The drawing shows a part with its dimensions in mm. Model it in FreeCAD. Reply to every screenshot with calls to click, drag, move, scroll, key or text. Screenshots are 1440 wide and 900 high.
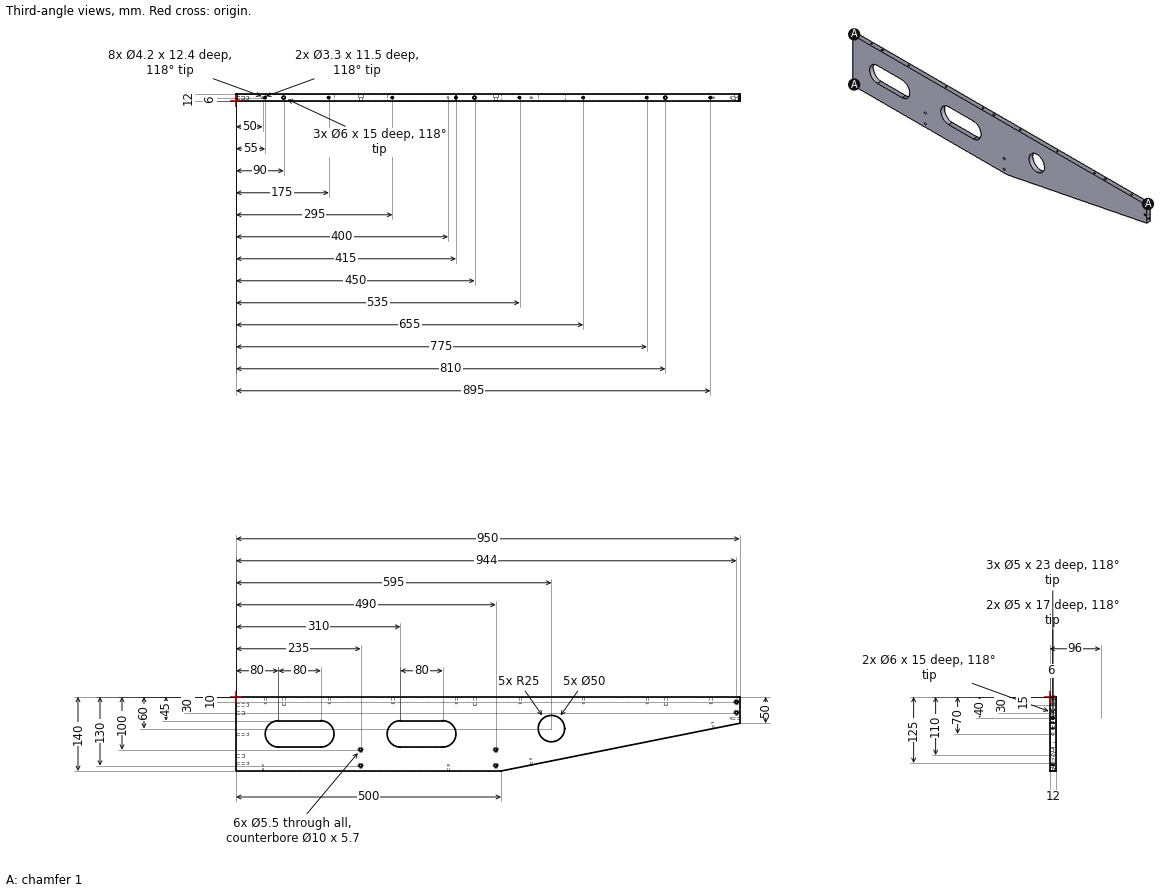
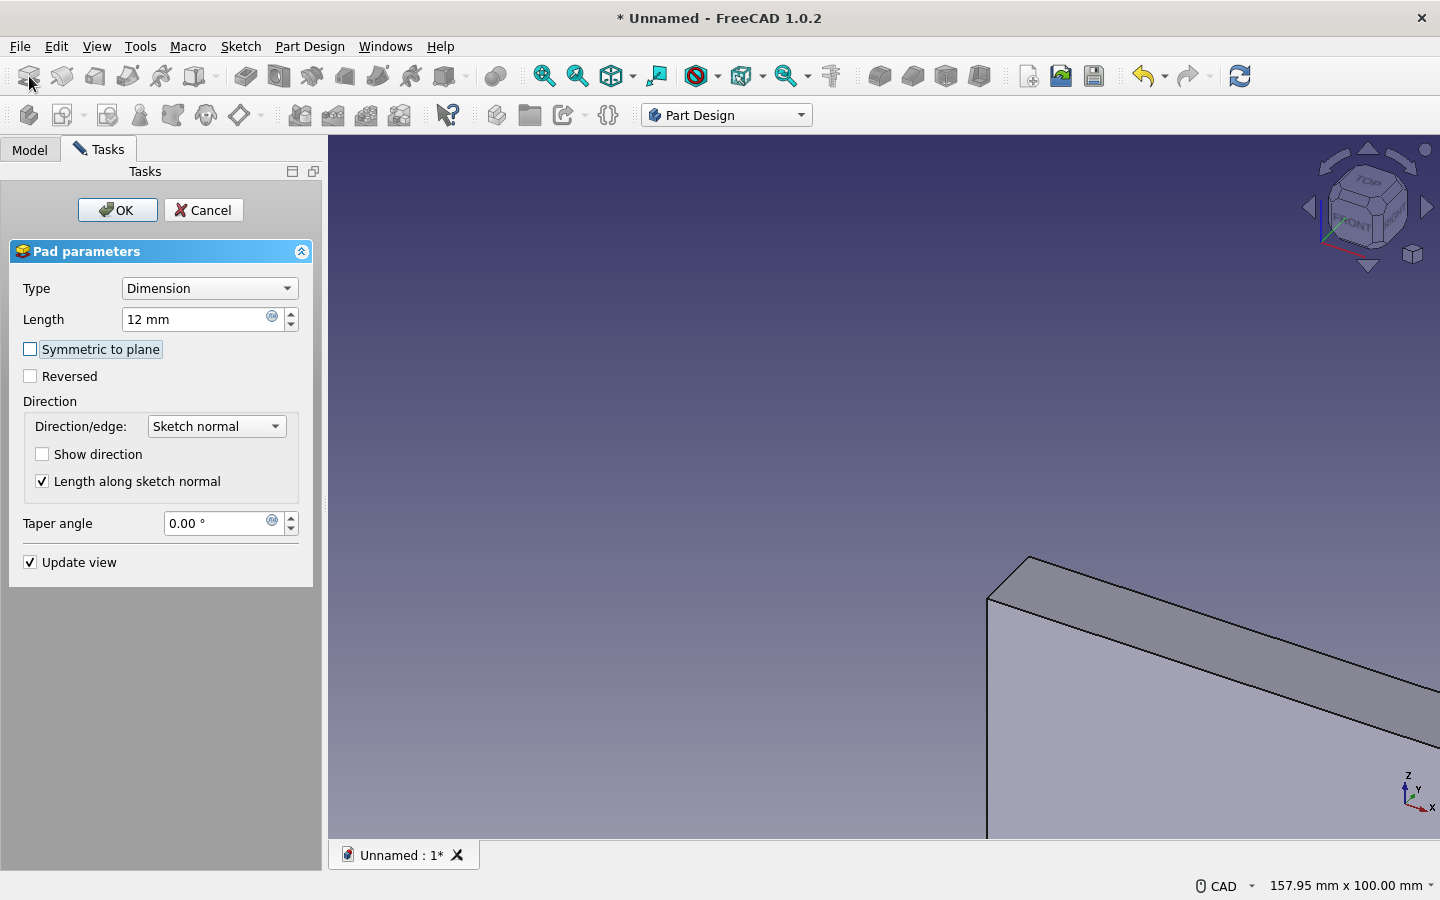
click(31, 376)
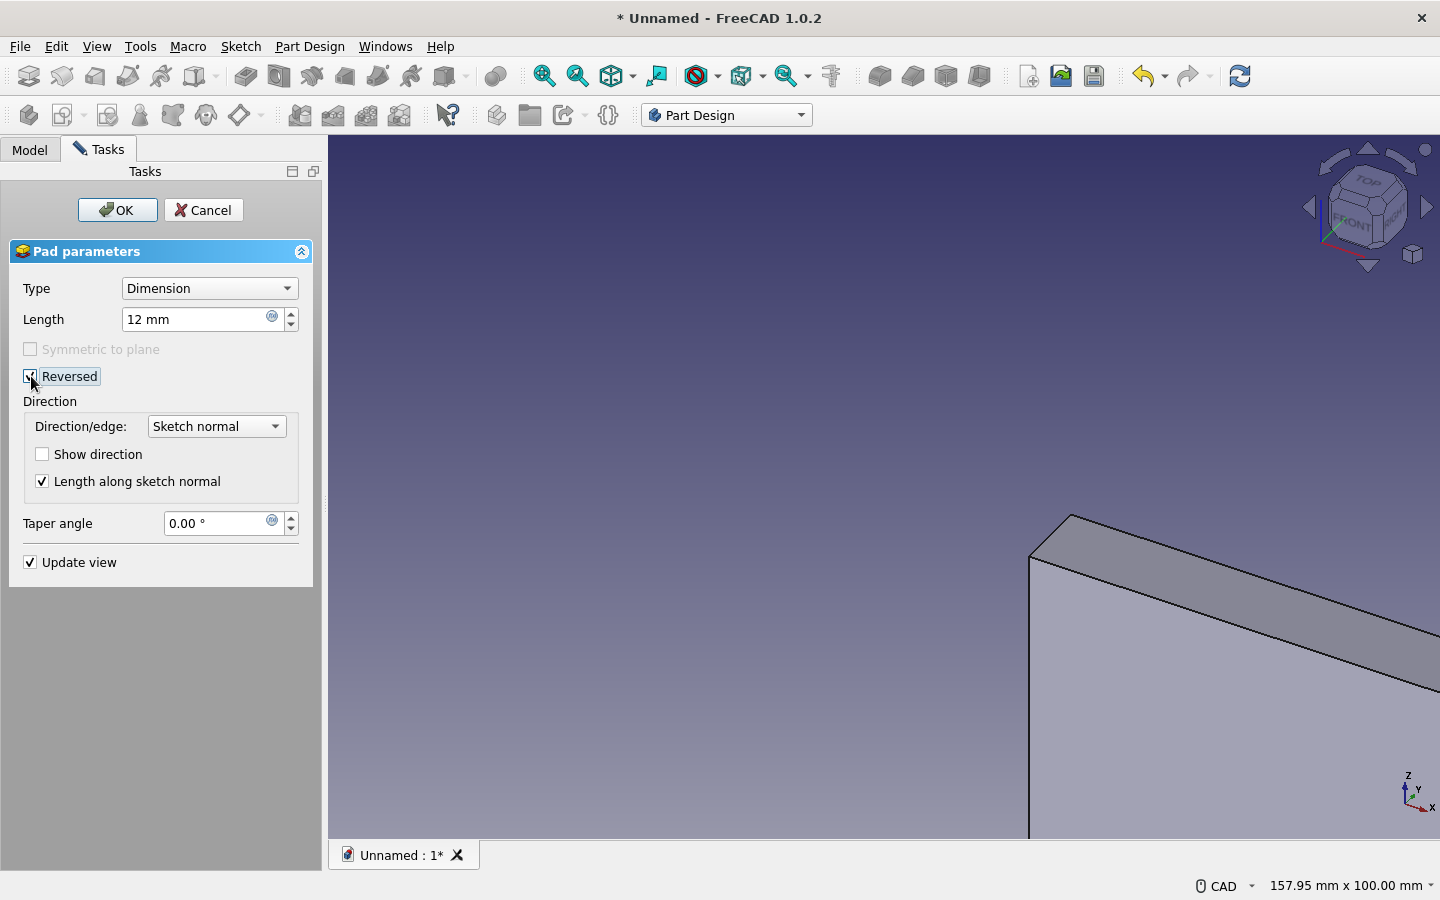
click(118, 210)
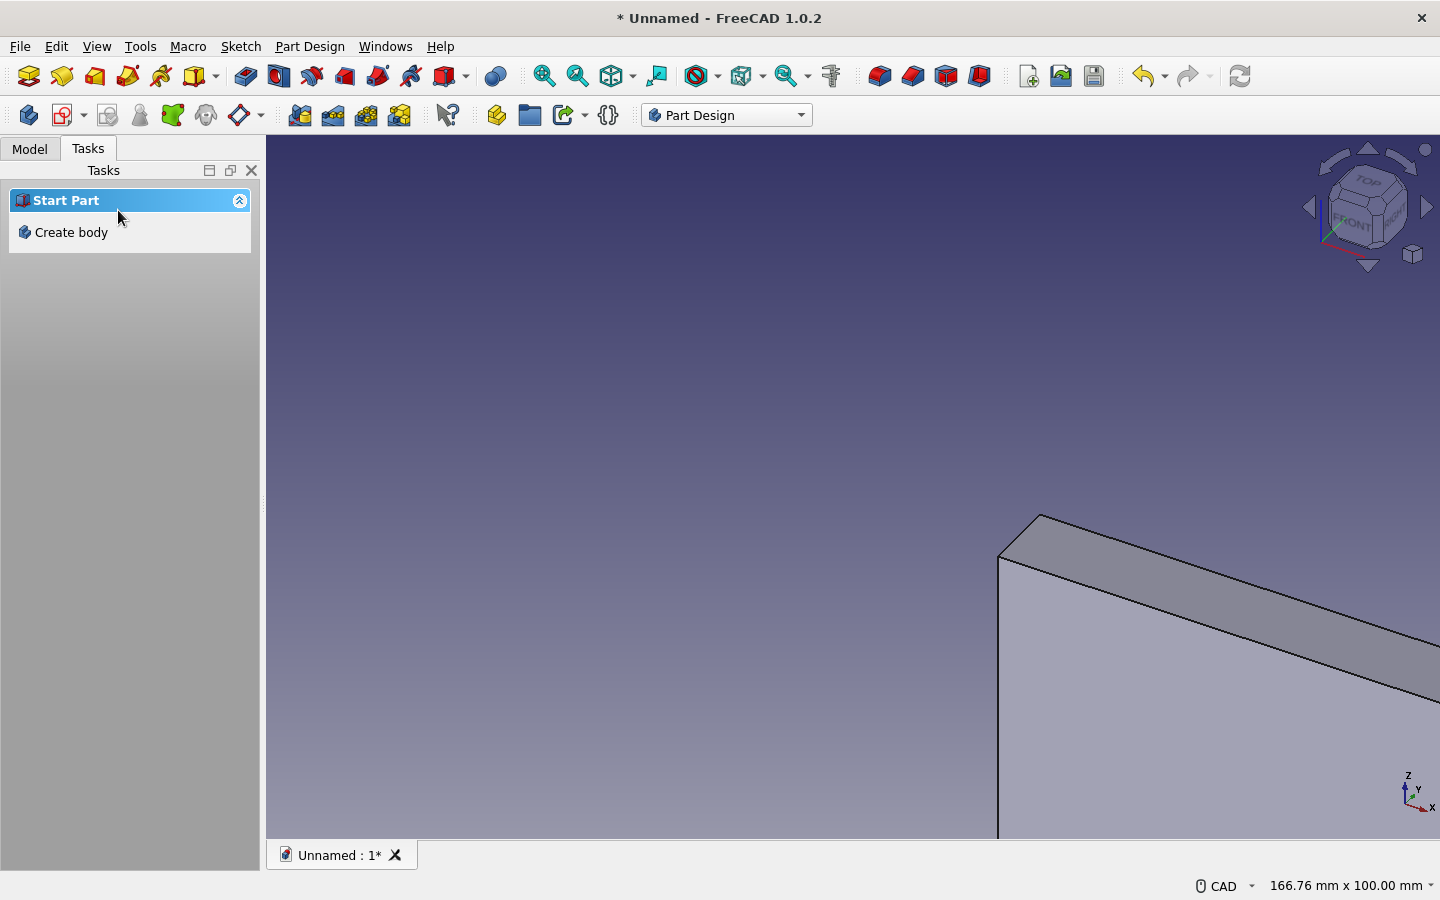
click(545, 76)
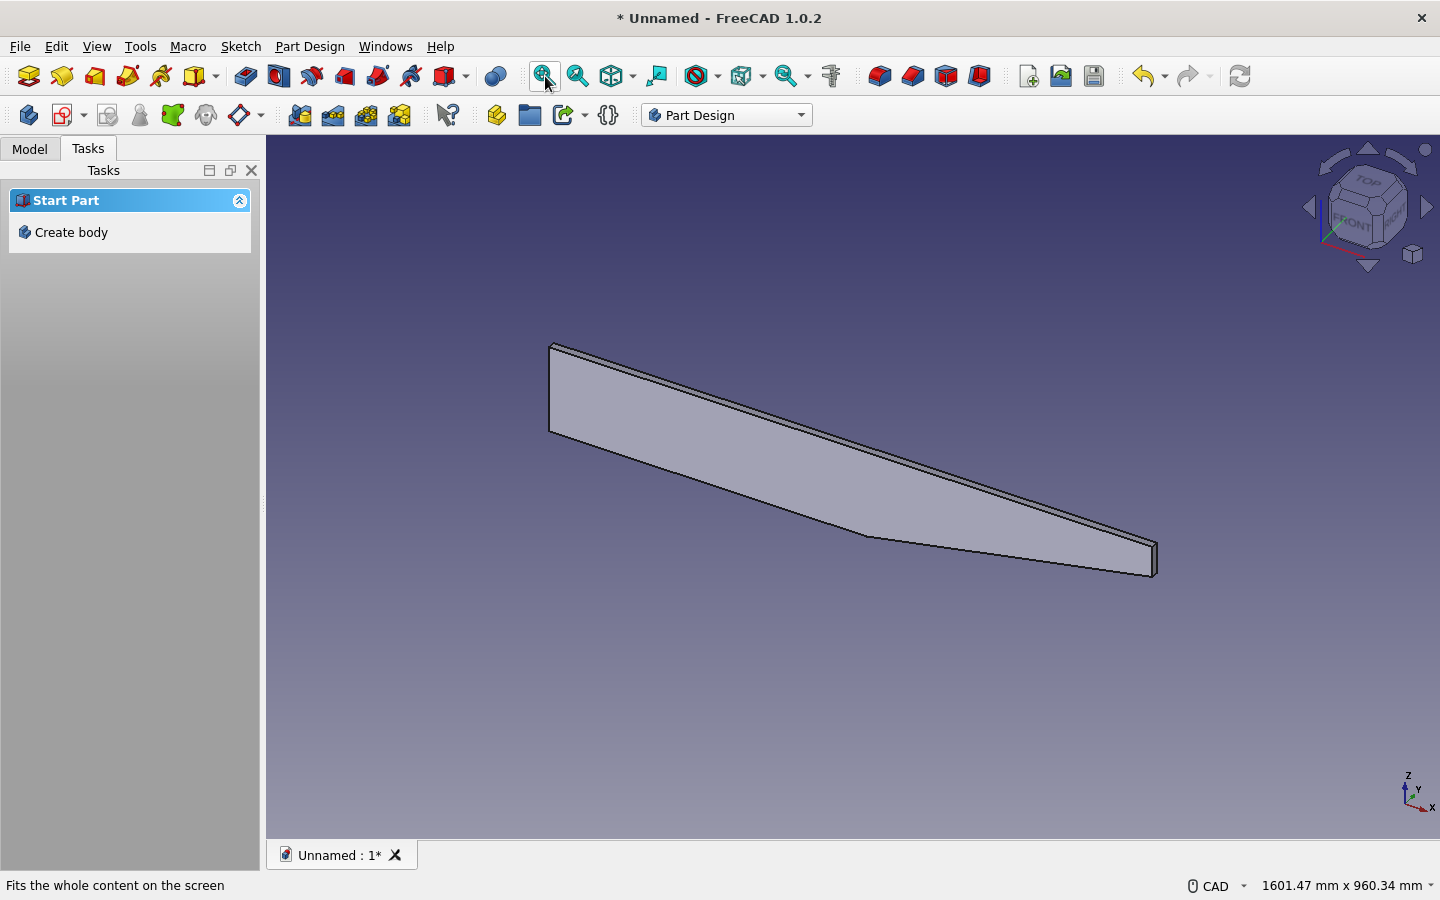
click(62, 116)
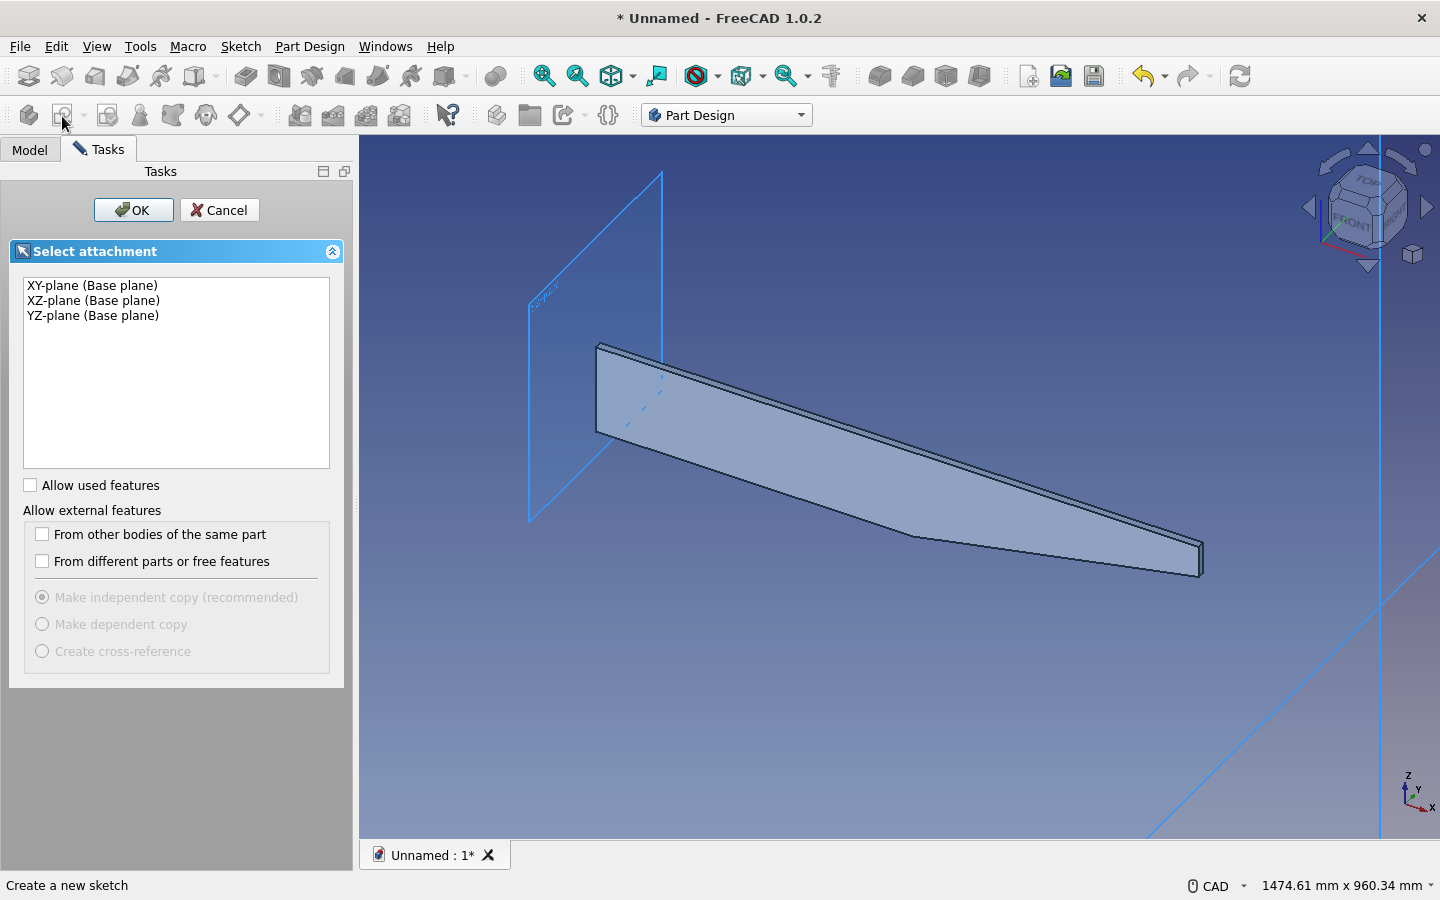
click(84, 300)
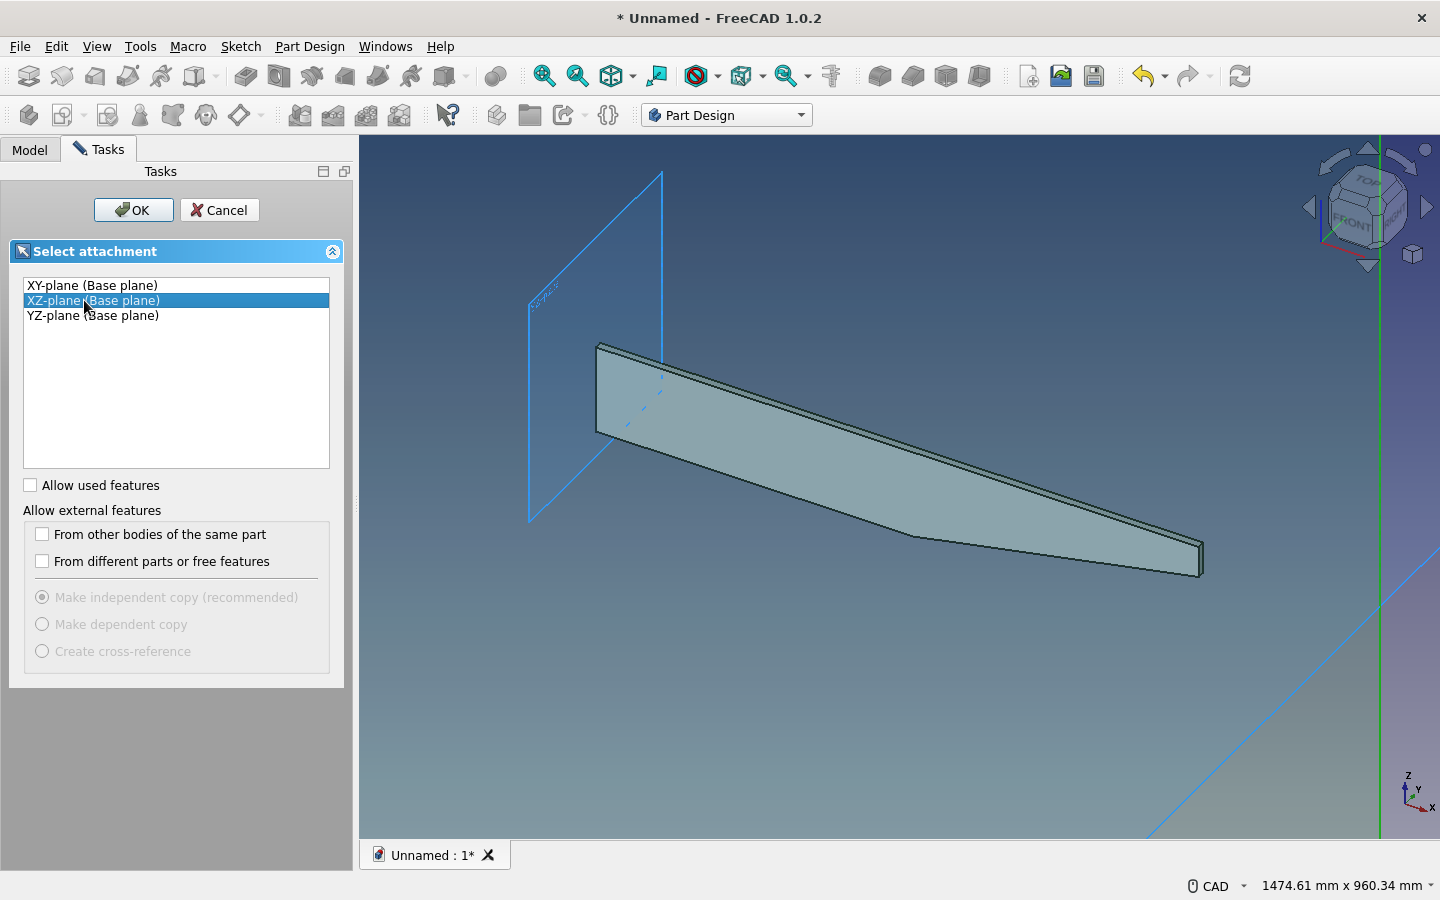
click(134, 210)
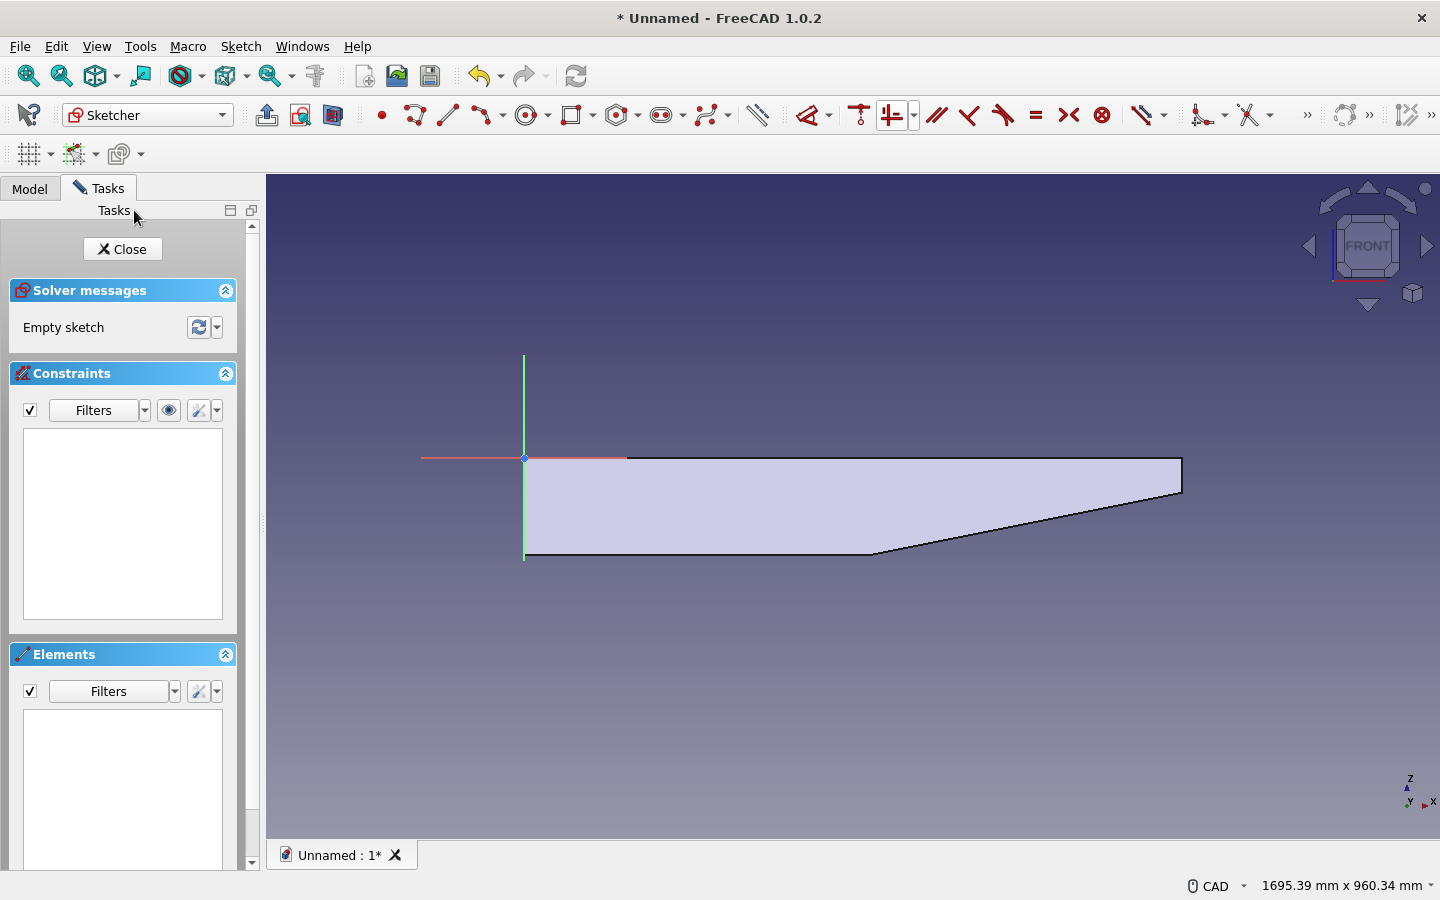
scroll(646, 459, up, 2)